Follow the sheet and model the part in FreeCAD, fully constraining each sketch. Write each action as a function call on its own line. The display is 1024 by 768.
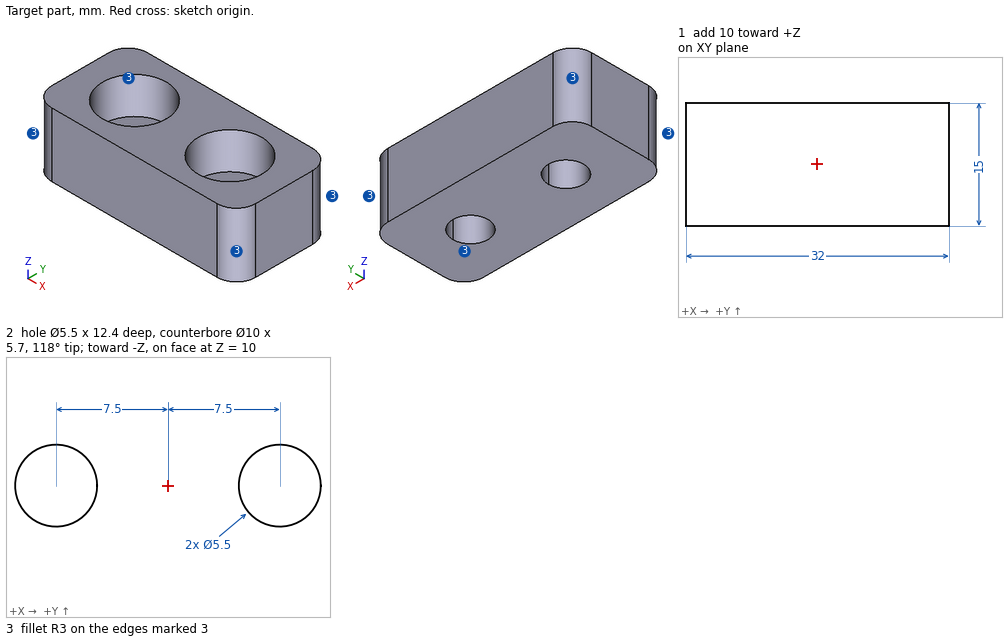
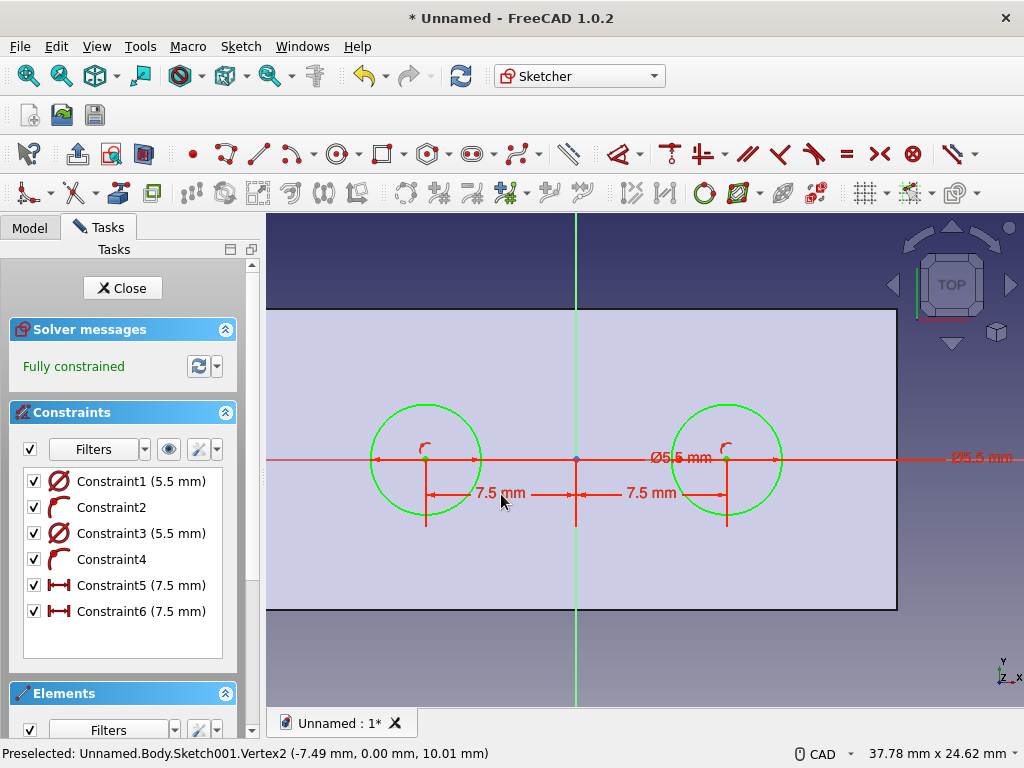
click(123, 288)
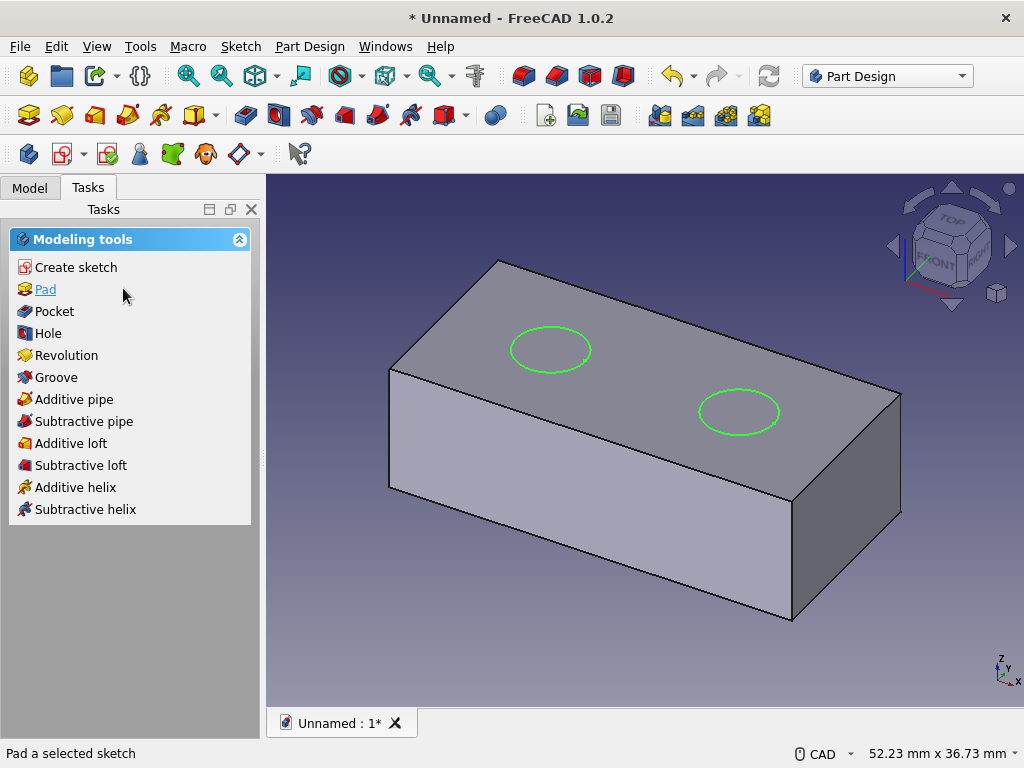
click(279, 116)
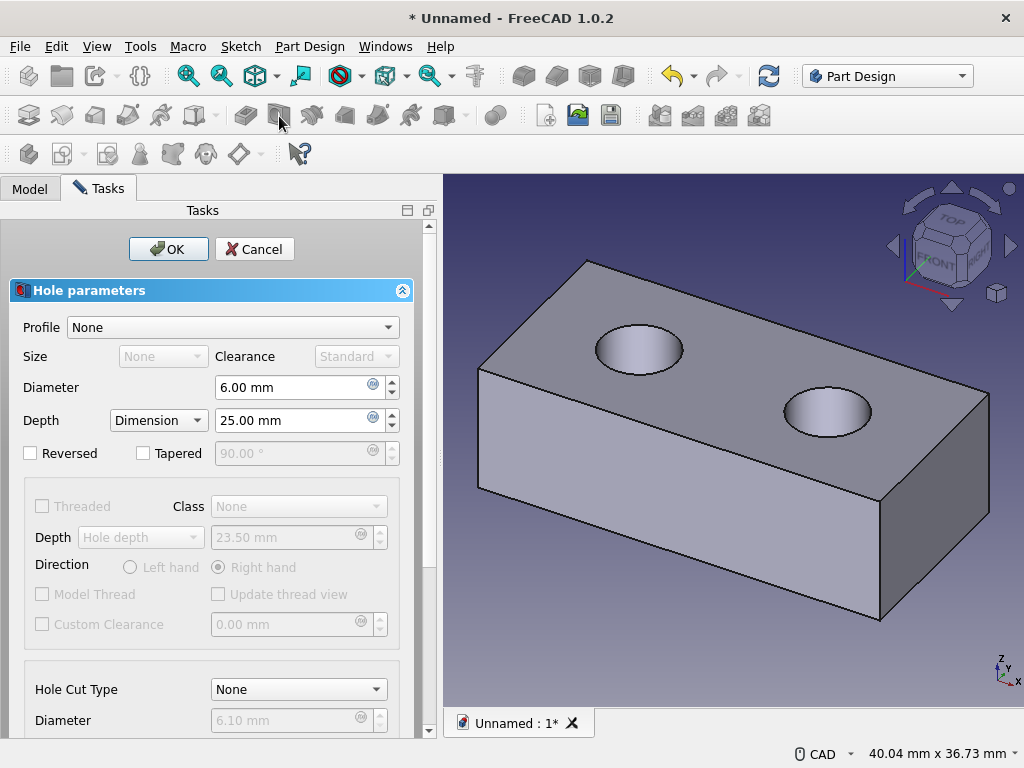
triple_click(300, 388)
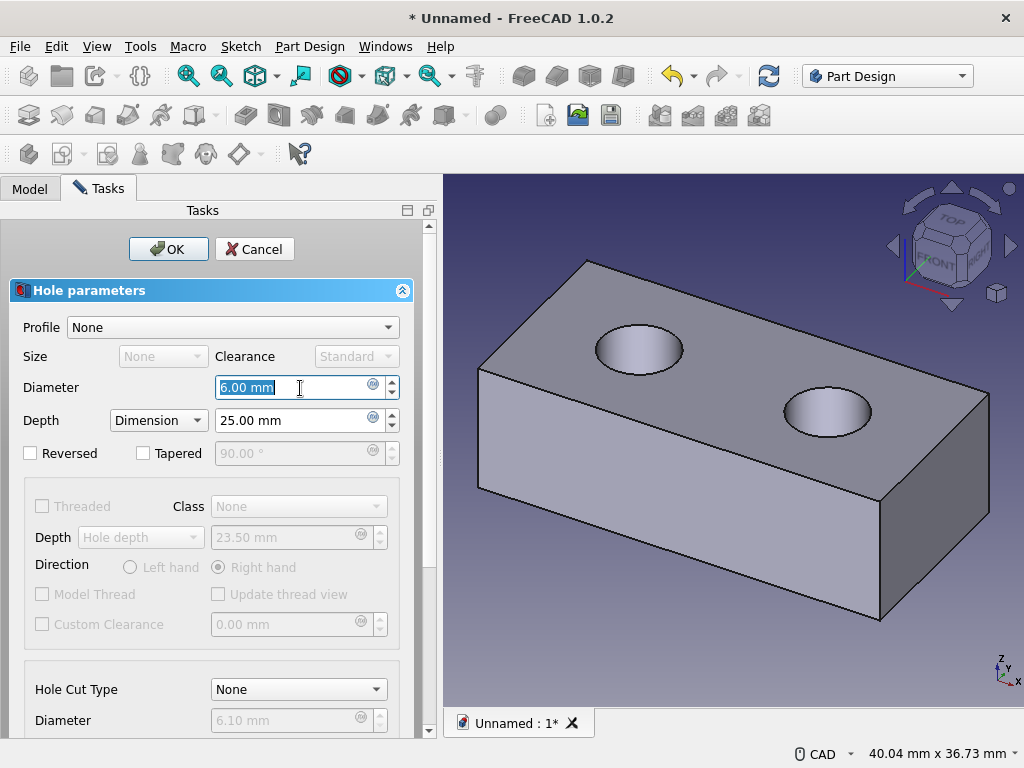
text(5.5)
key(Tab)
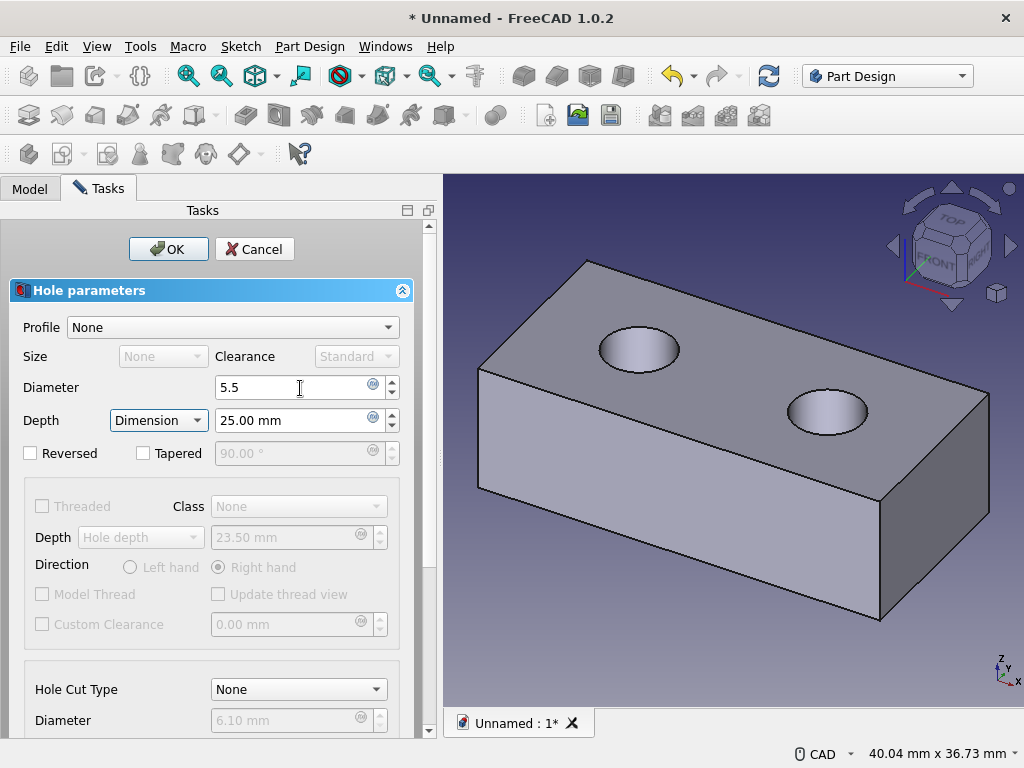
triple_click(300, 420)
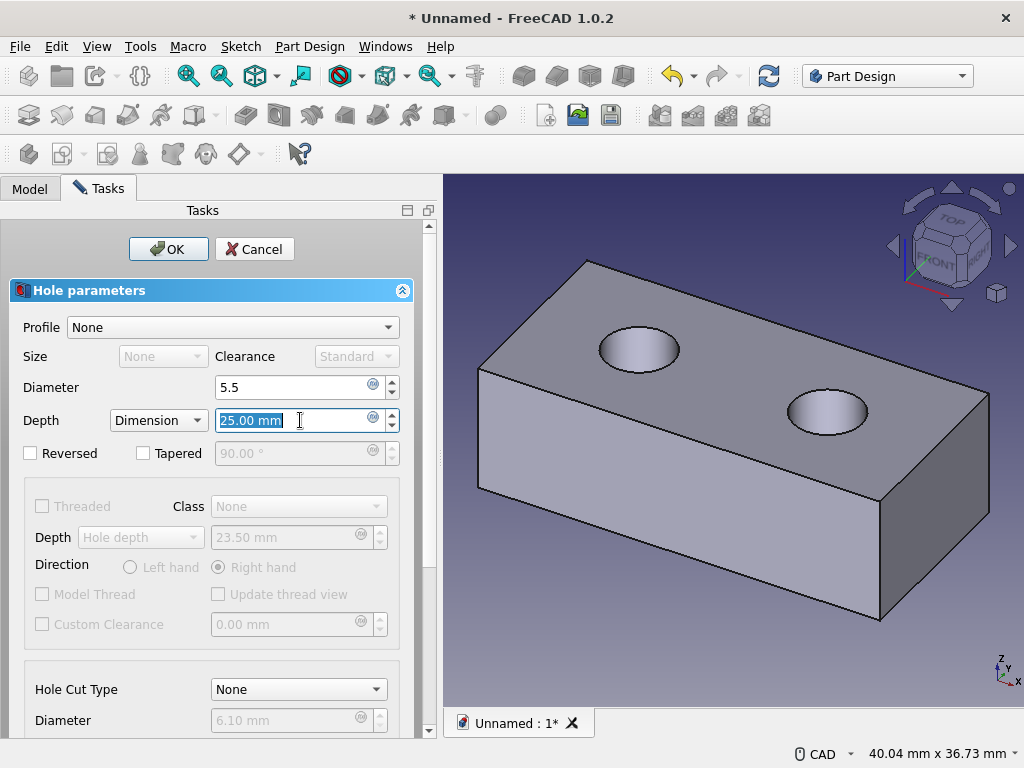
text(12.4)
key(Tab)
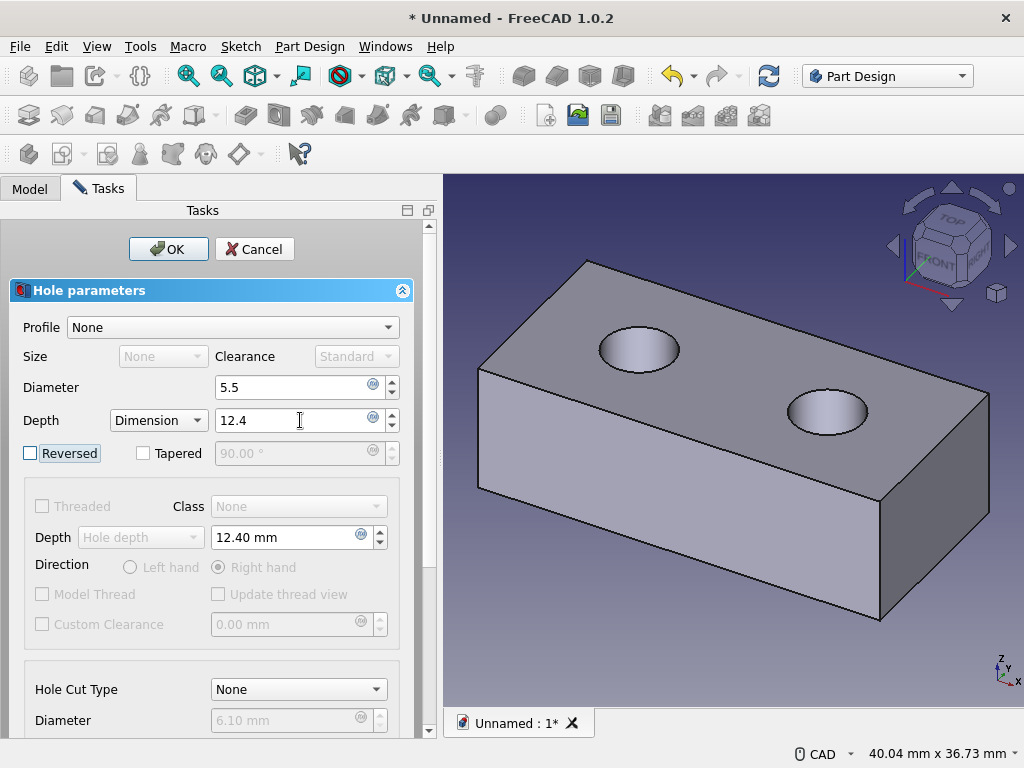
click(300, 690)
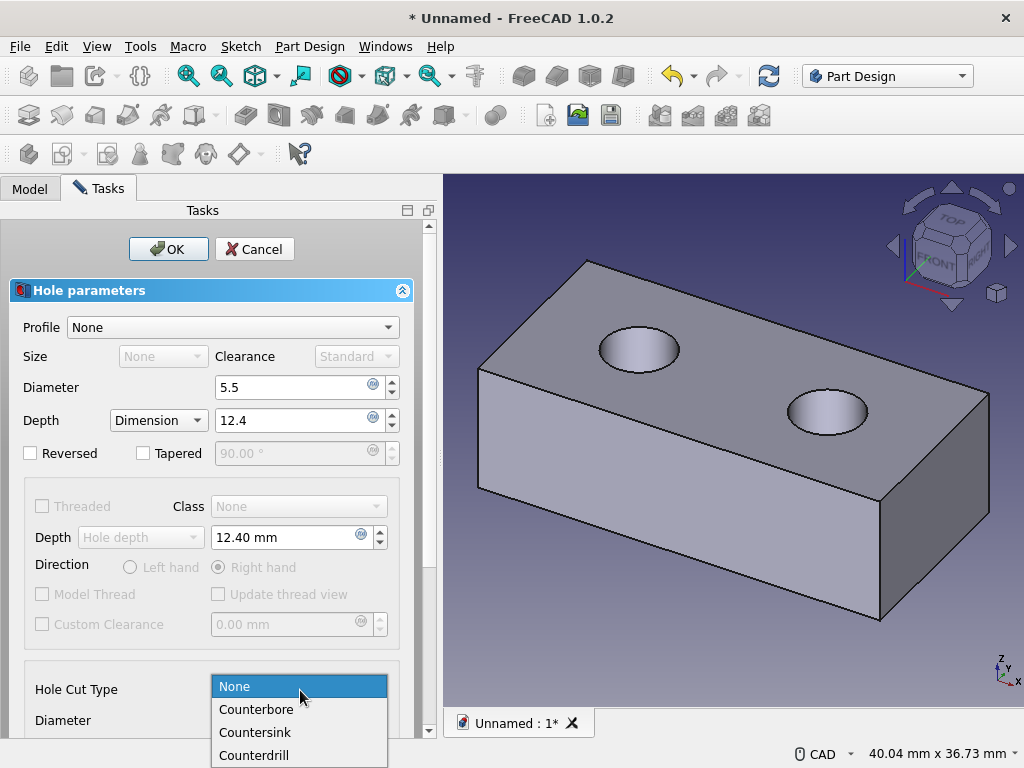
click(298, 710)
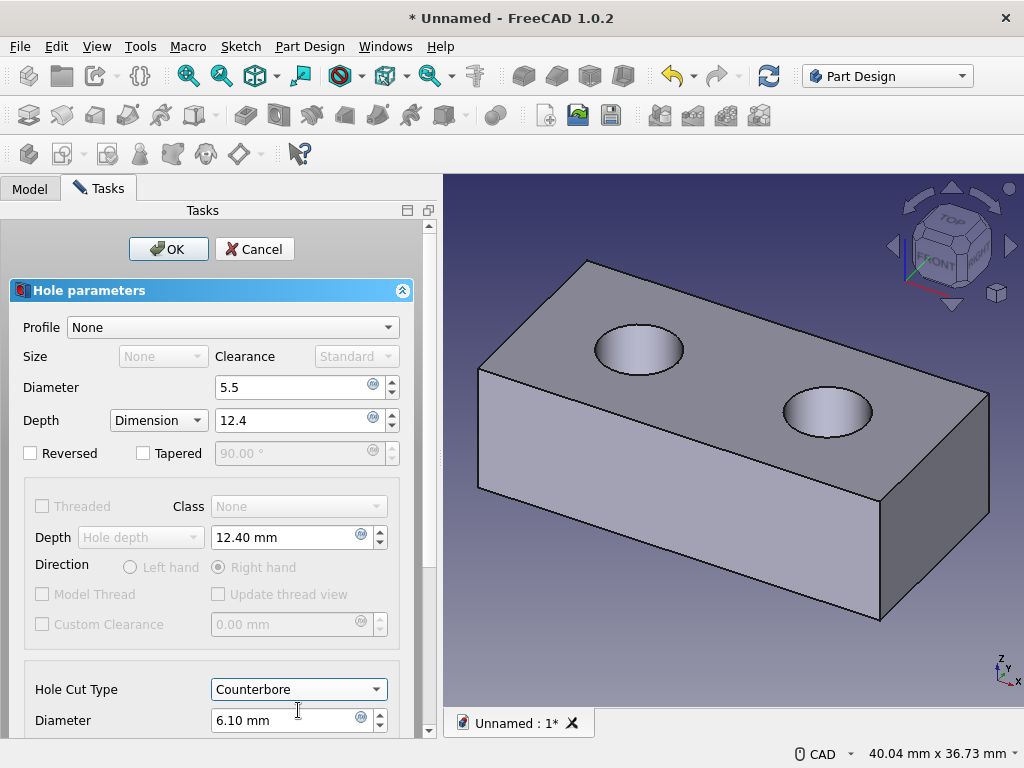
triple_click(292, 720)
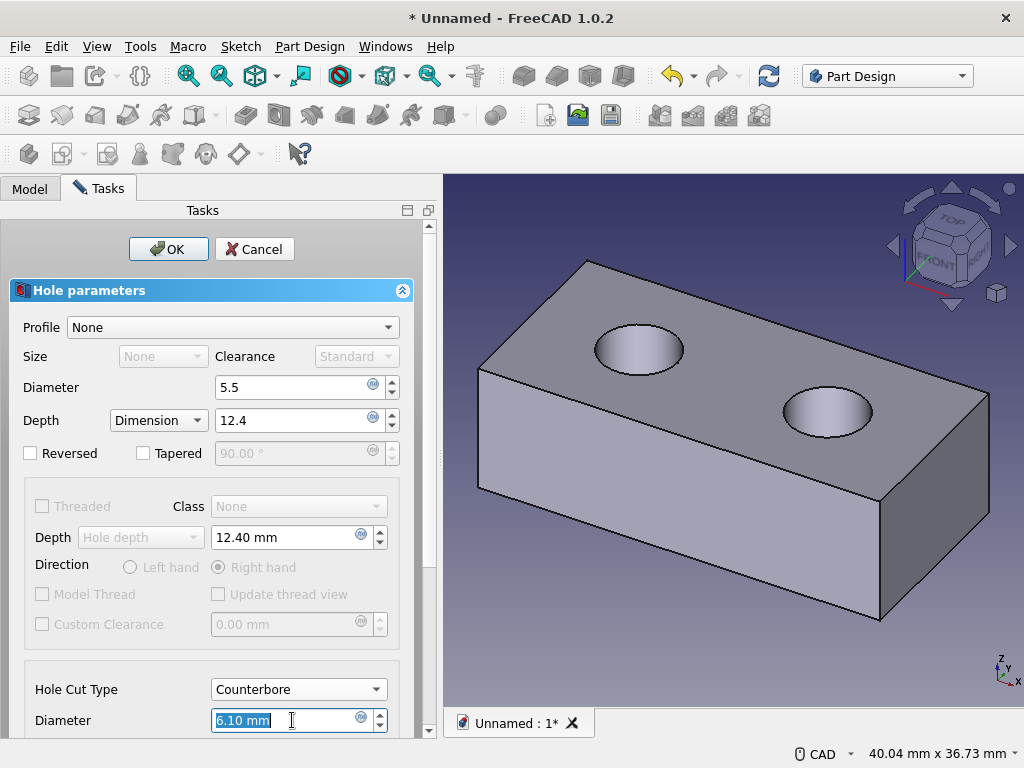
text(10)
key(Tab)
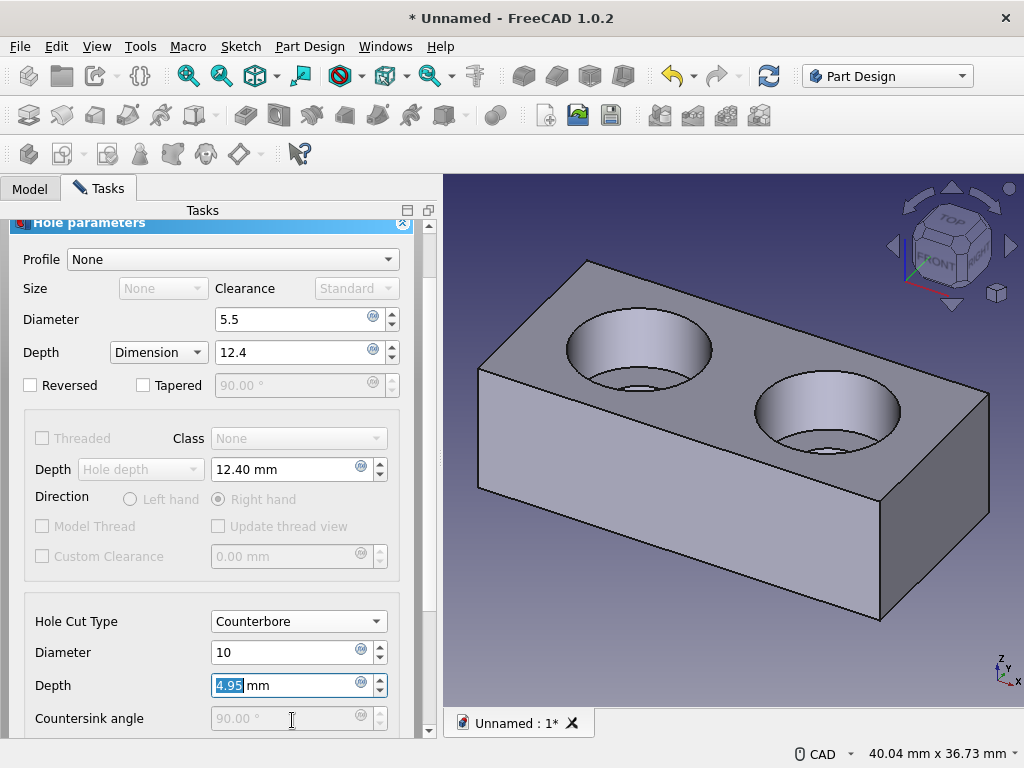
text(5.7)
key(Tab)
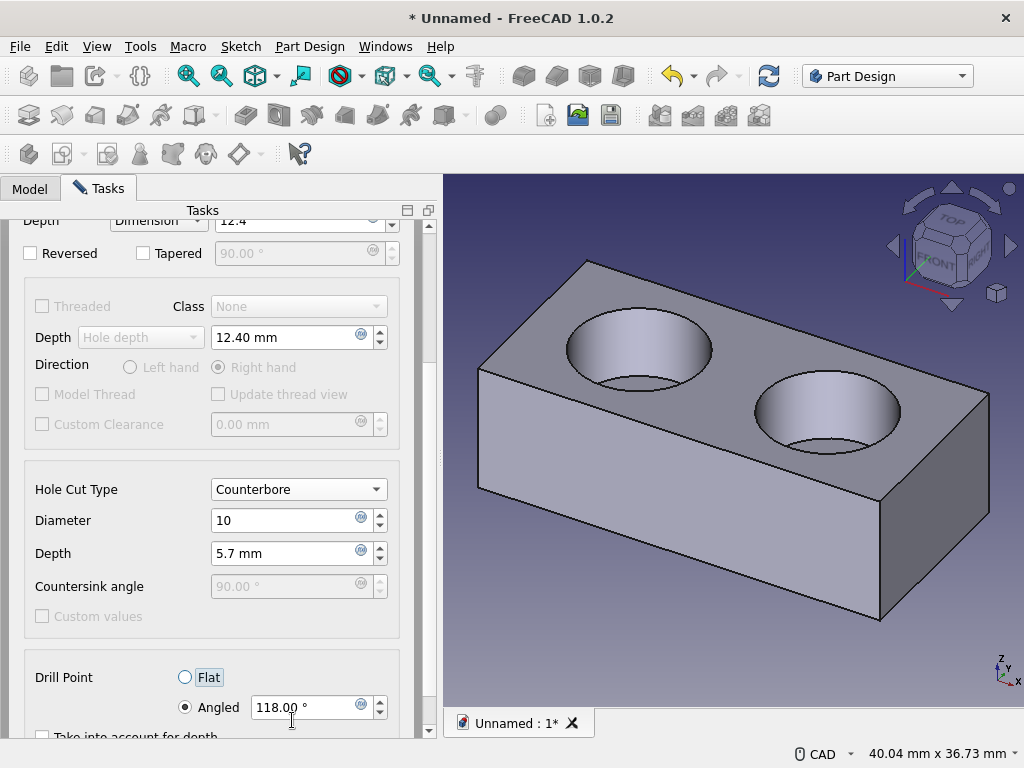
scroll(429, 479, up, 5)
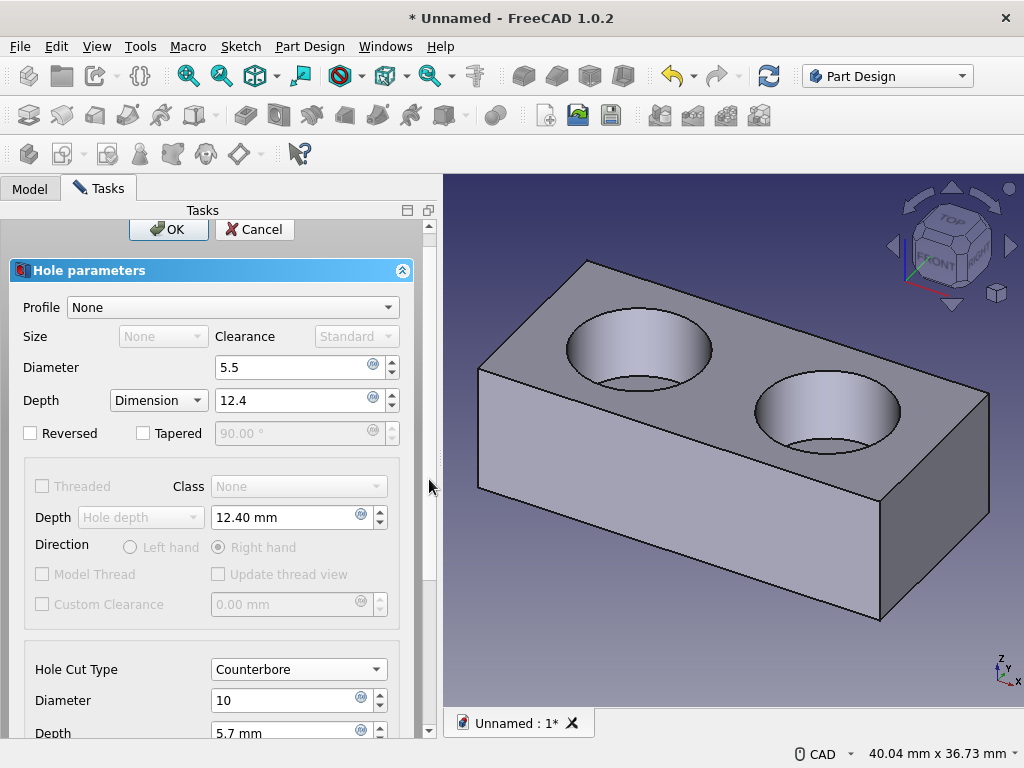
click(169, 249)